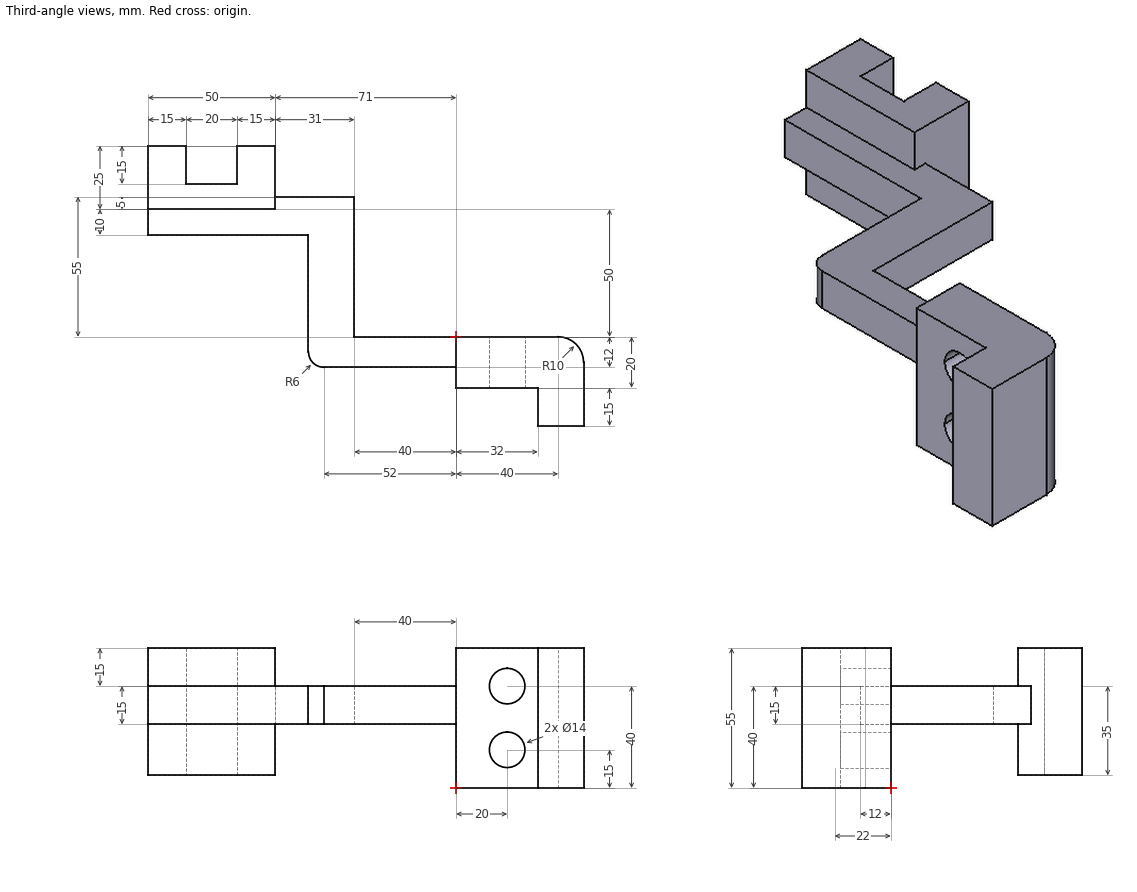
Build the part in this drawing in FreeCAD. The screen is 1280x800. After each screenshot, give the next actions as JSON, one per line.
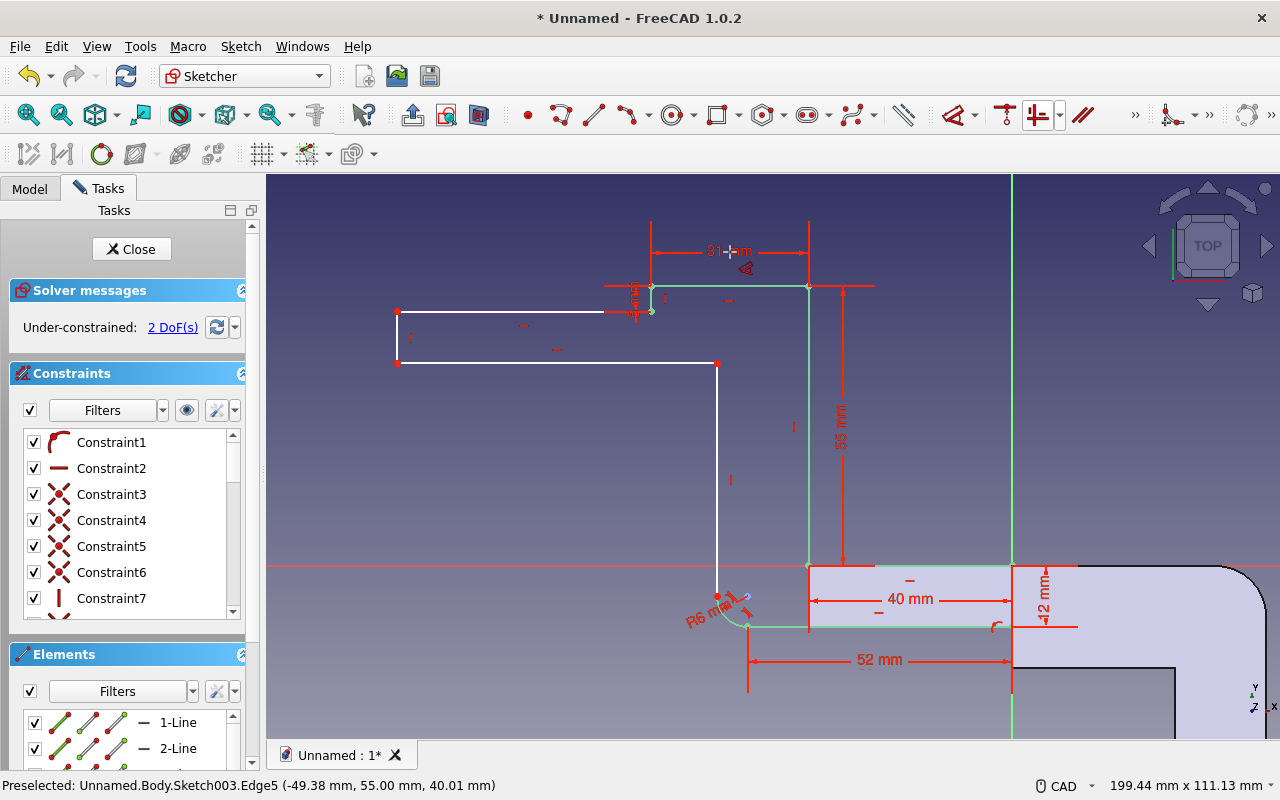
{"action": "left_click", "coordinate": [575, 312]}
{"action": "left_click", "coordinate": [524, 278]}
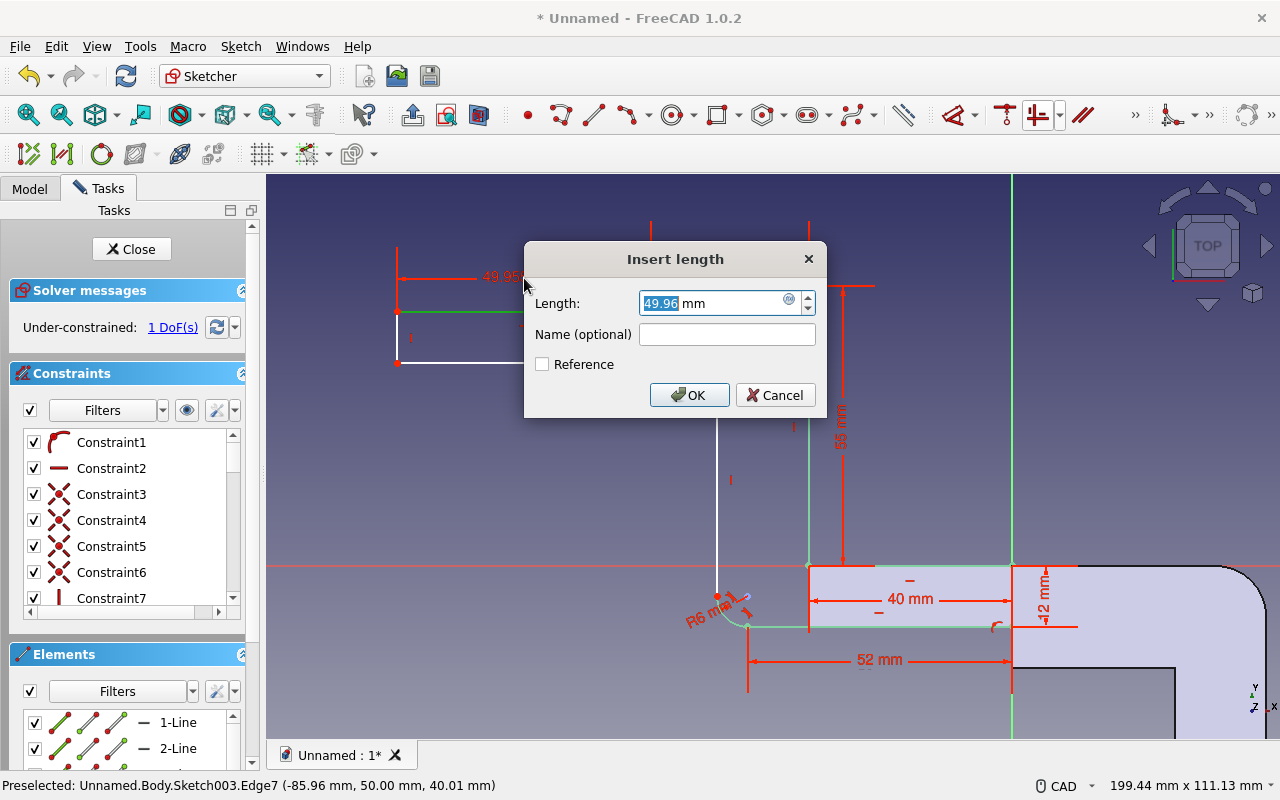
{"action": "type", "text": "50"}
{"action": "key", "text": "Return"}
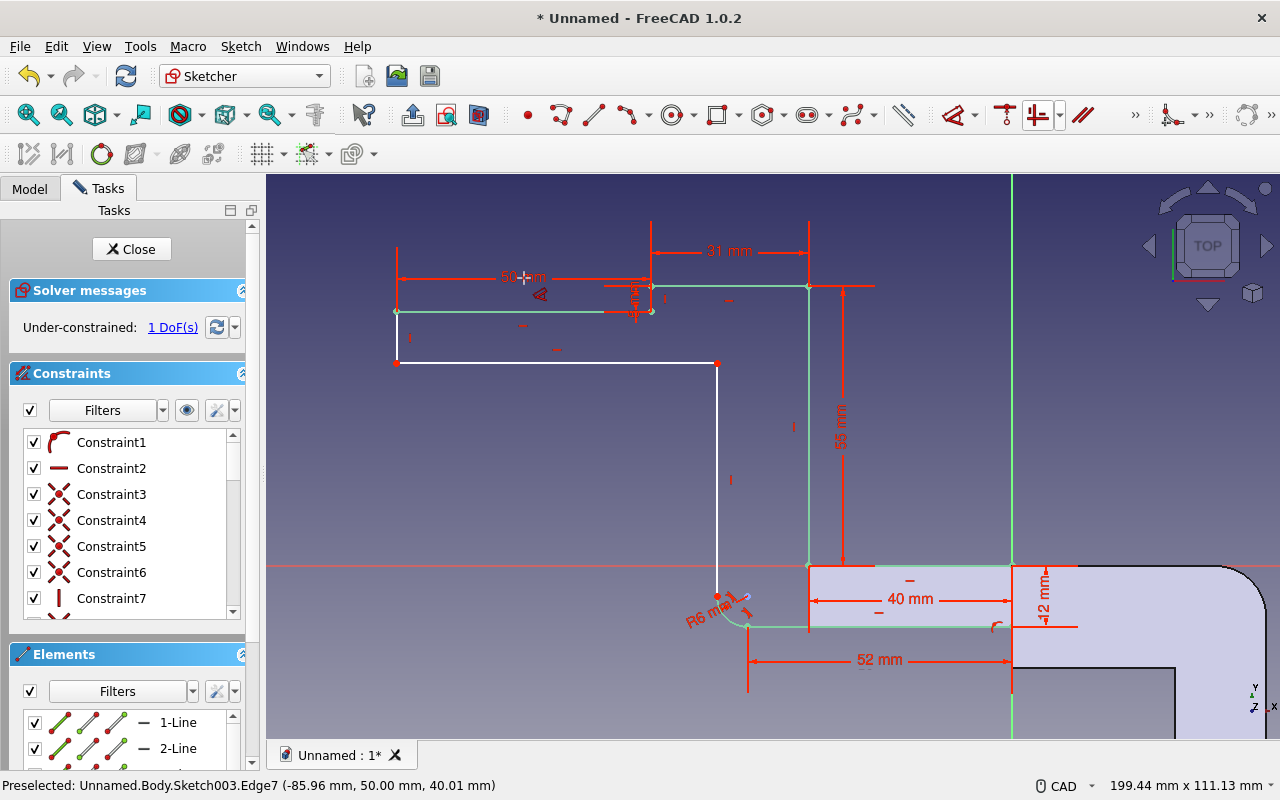
{"action": "left_click", "coordinate": [397, 327]}
{"action": "left_click", "coordinate": [363, 337]}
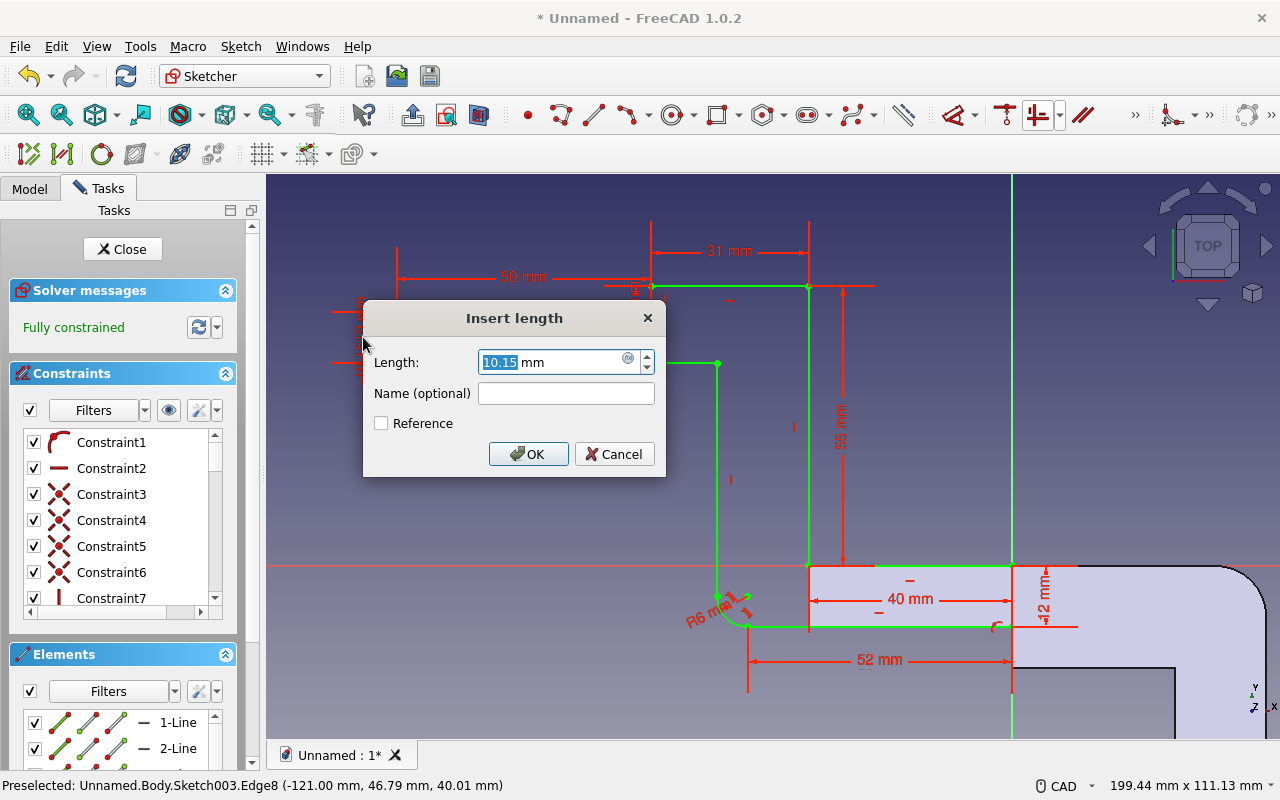
{"action": "type", "text": "10"}
{"action": "key", "text": "Return"}
{"action": "key", "text": "Escape"}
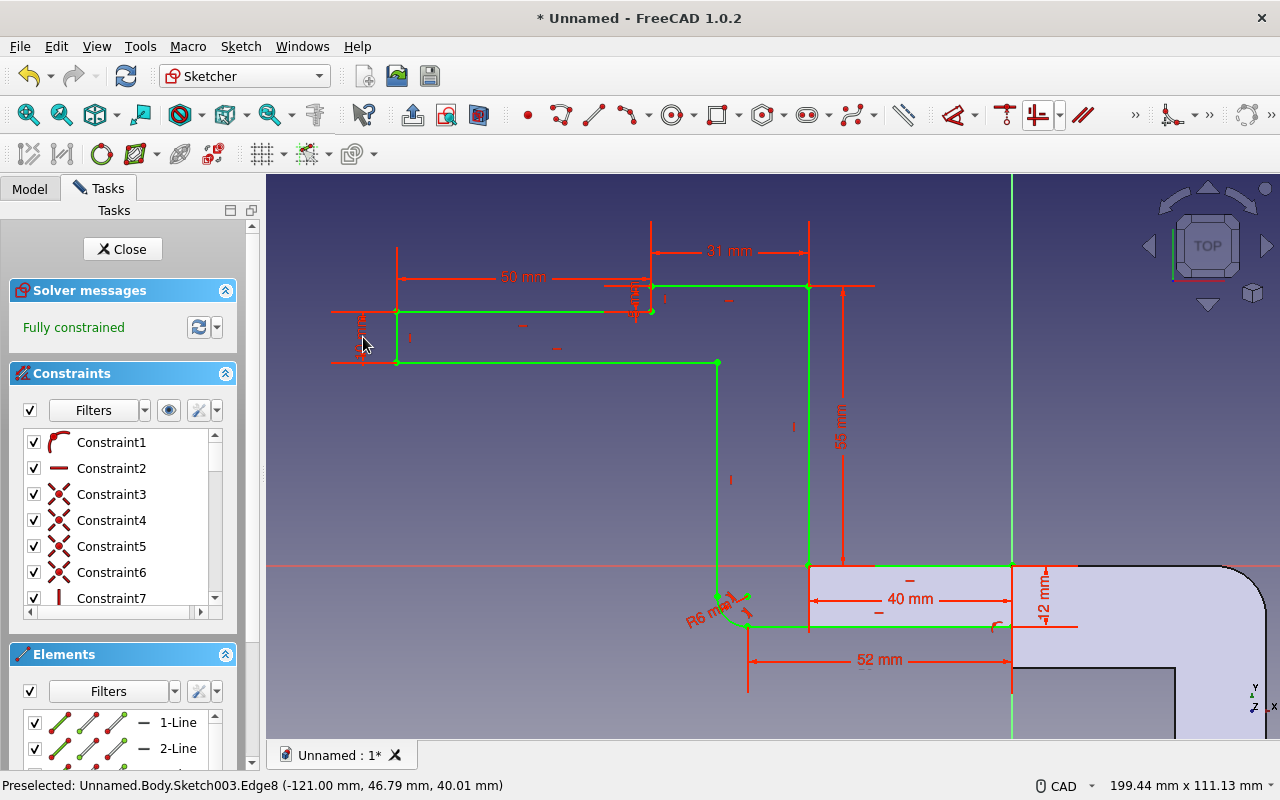
{"action": "left_click", "coordinate": [123, 249]}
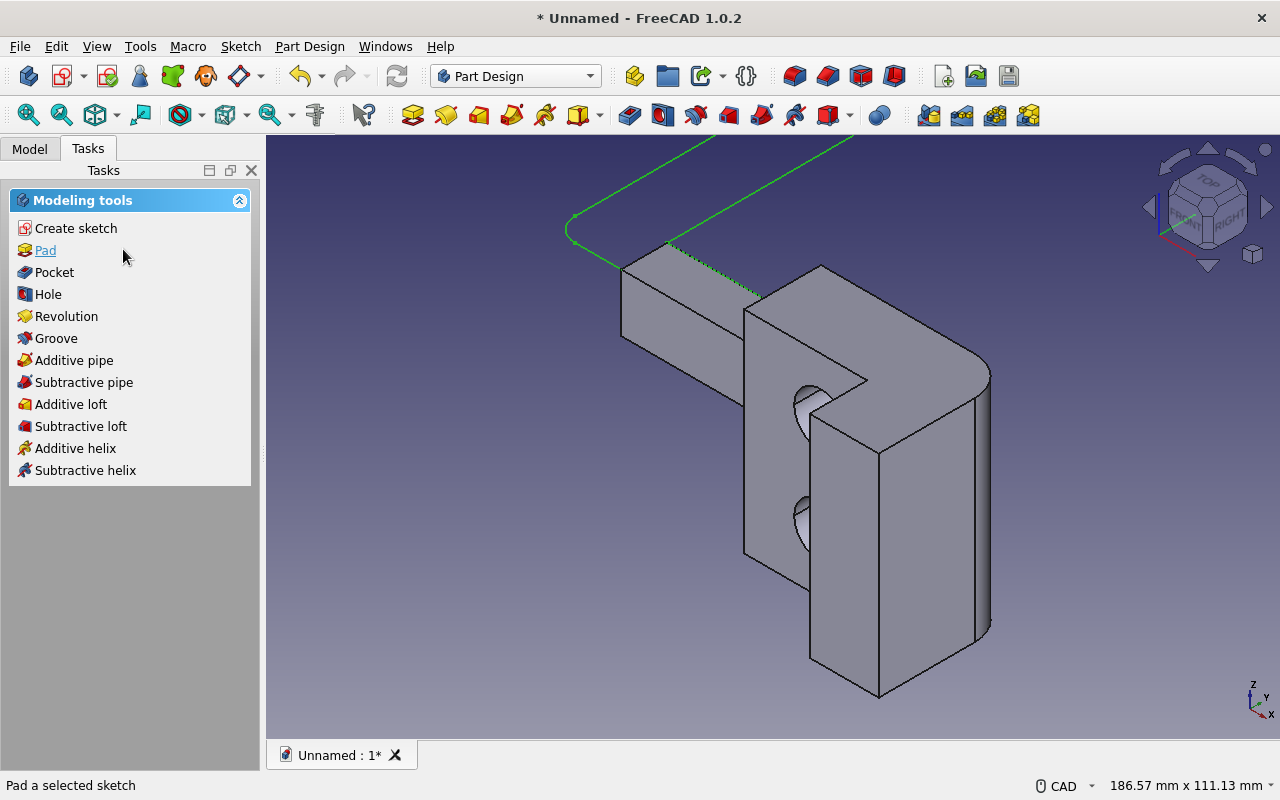
{"action": "left_click", "coordinate": [413, 116]}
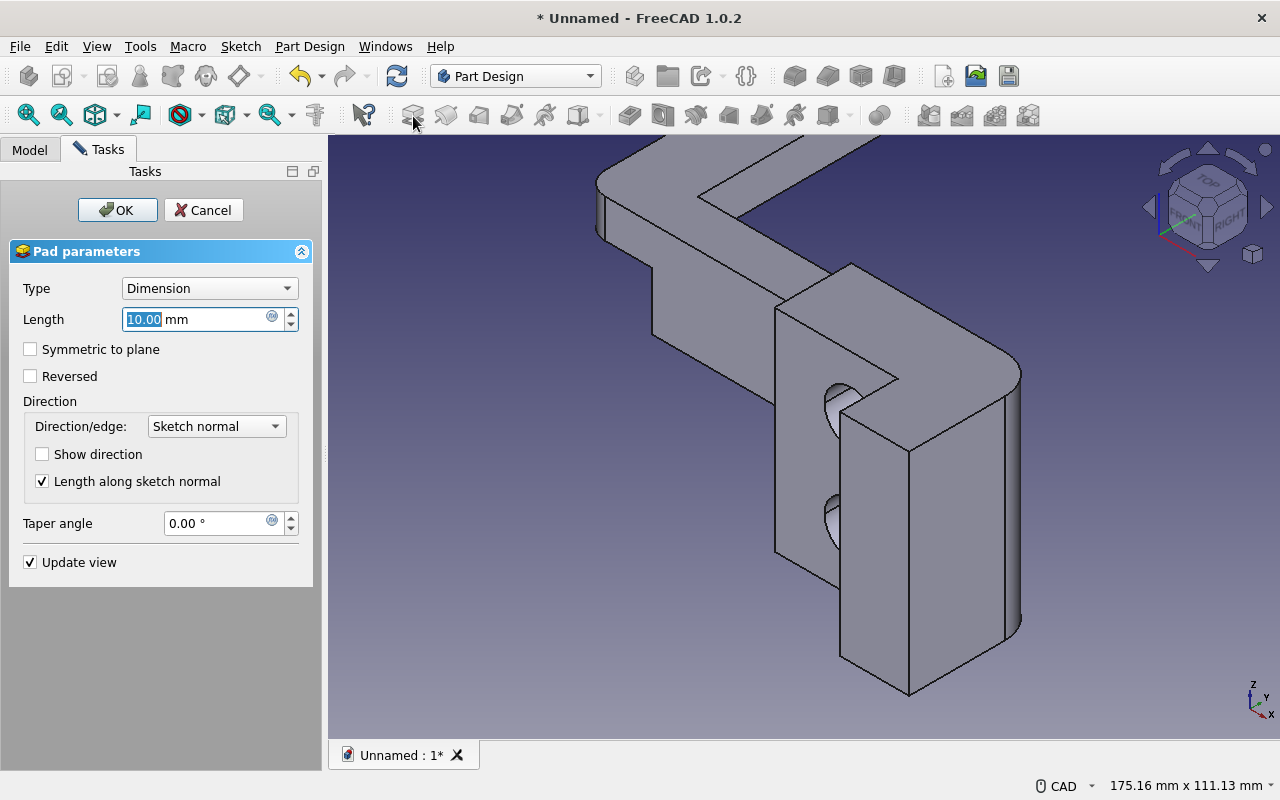
{"action": "type", "text": "15"}
{"action": "key", "text": "Tab"}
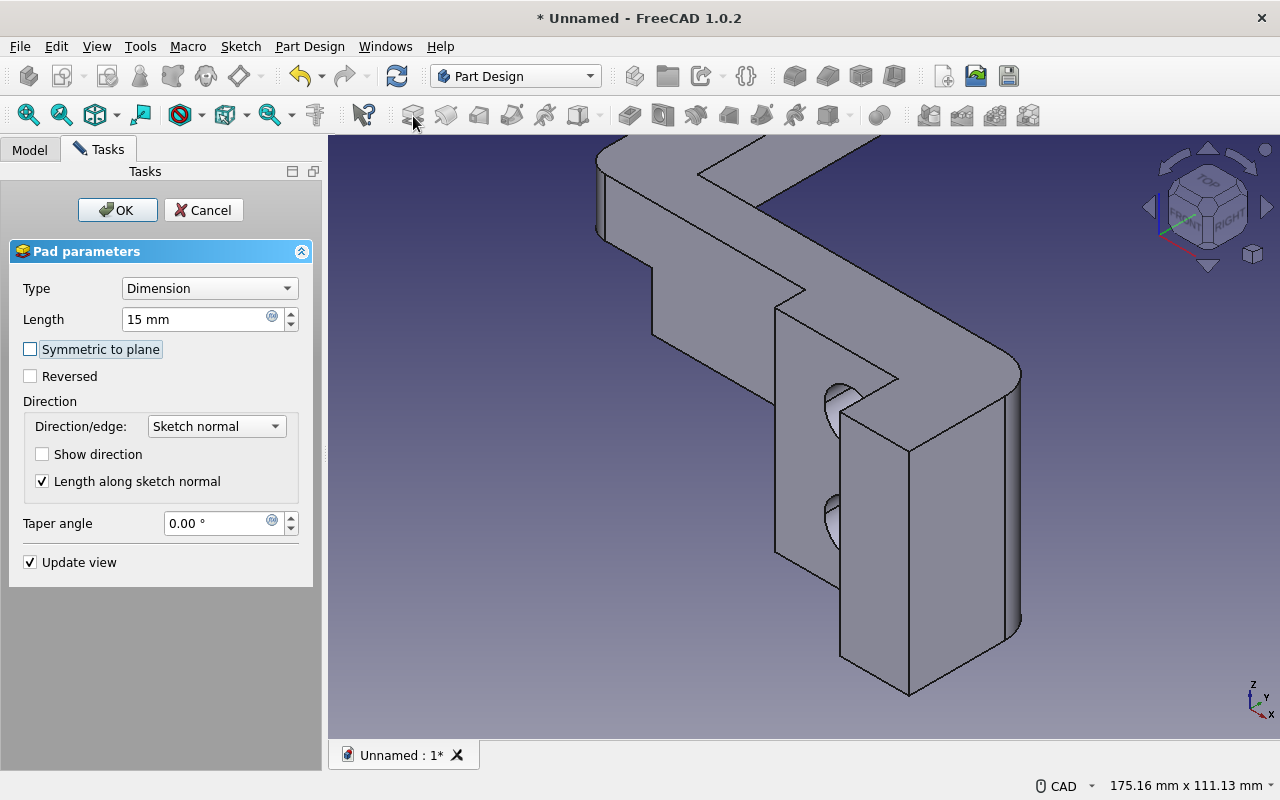
{"action": "left_click", "coordinate": [31, 376]}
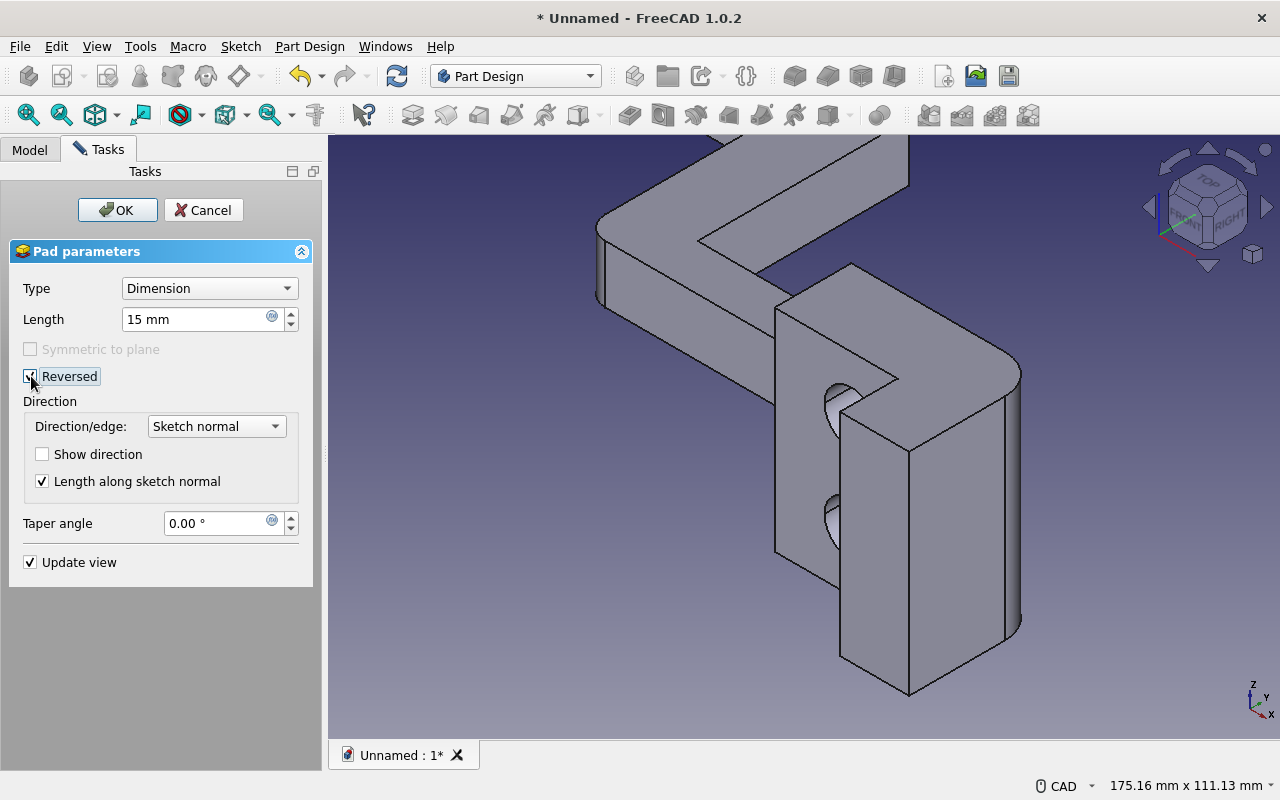
{"action": "left_click", "coordinate": [118, 210]}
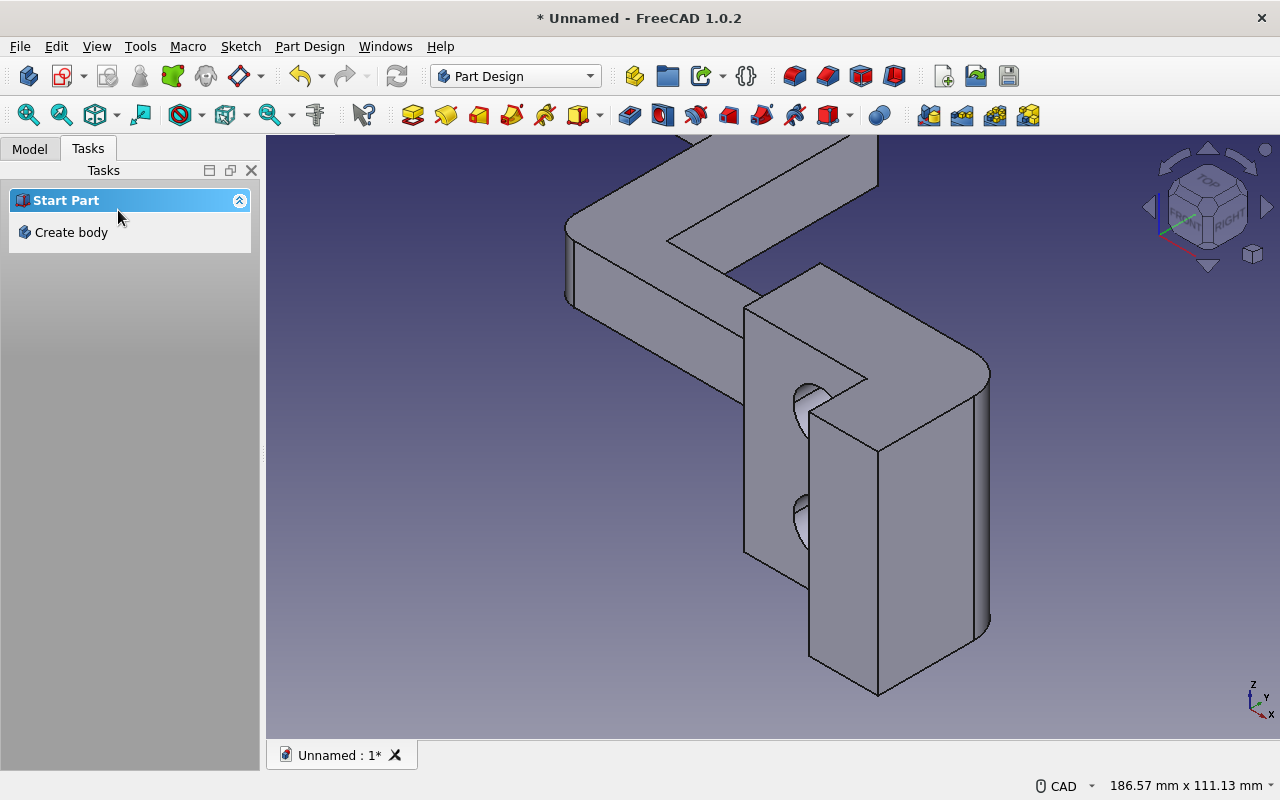
{"action": "left_click", "coordinate": [29, 116]}